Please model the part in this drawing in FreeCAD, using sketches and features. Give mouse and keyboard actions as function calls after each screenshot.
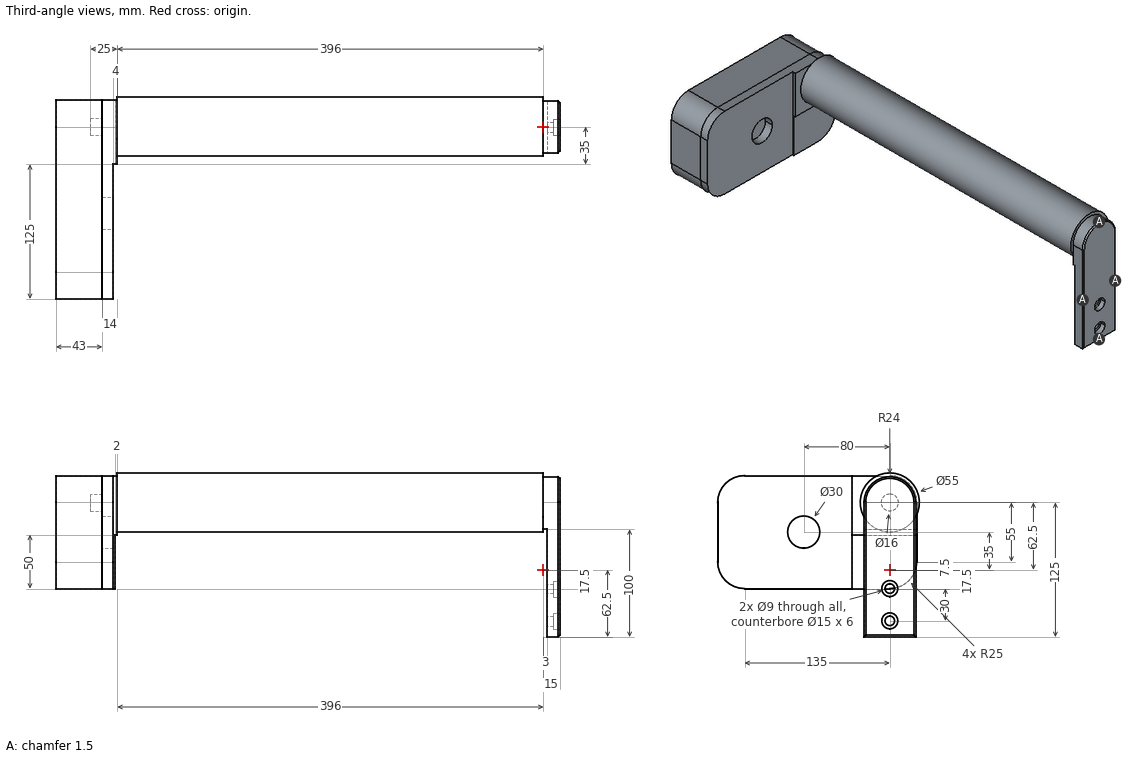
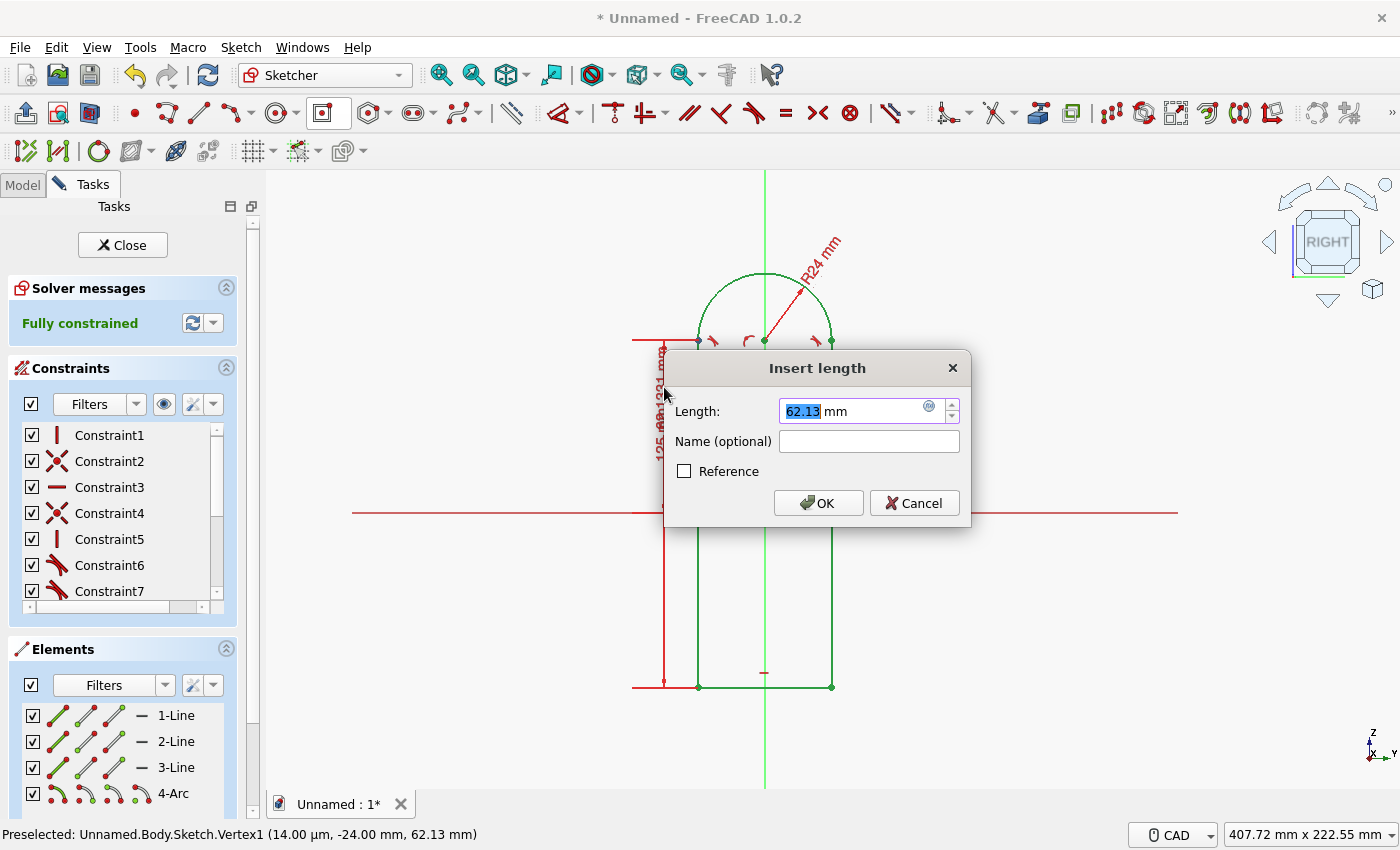
text(62.5)
key(Return)
key(Escape)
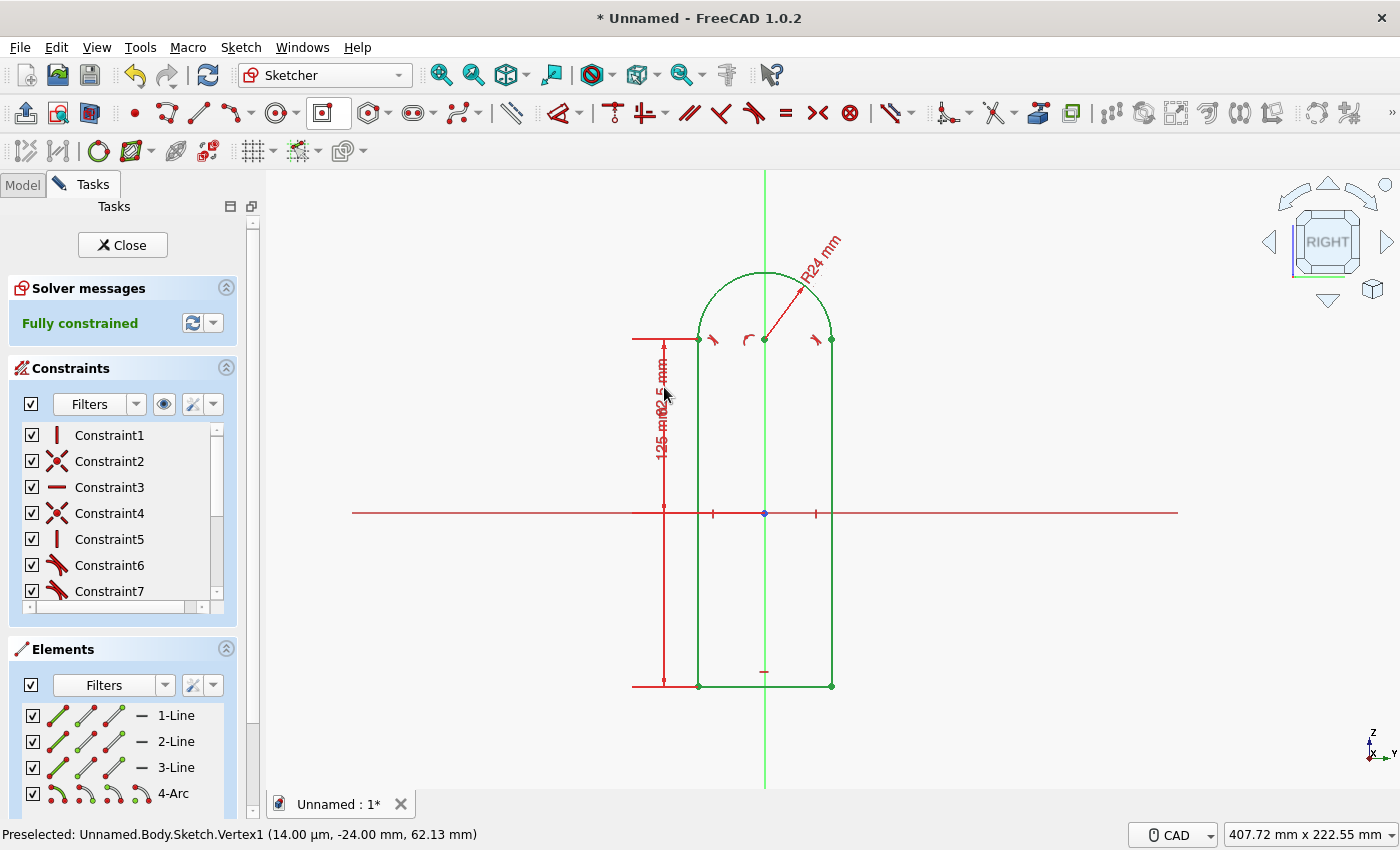
click(123, 245)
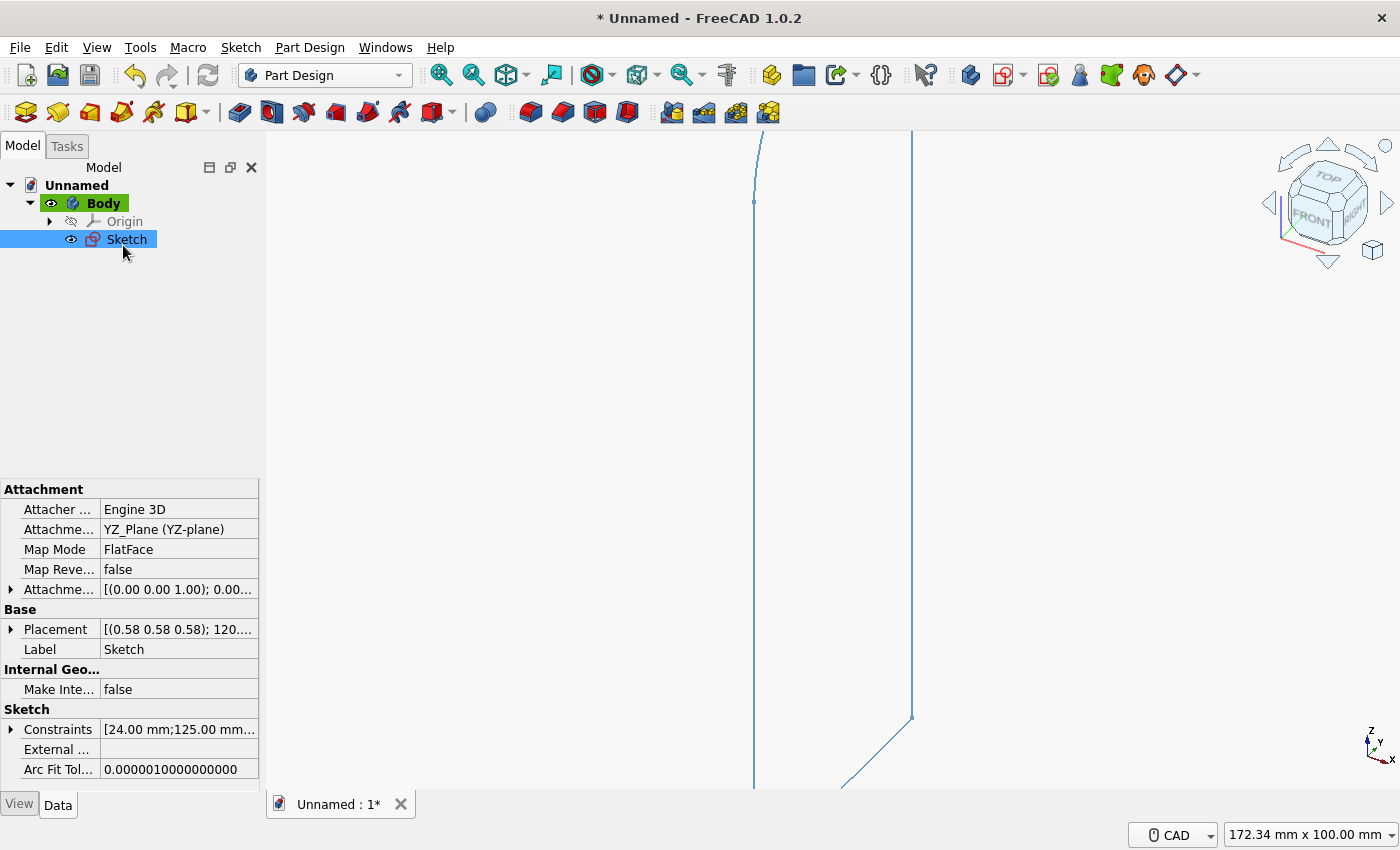
click(26, 112)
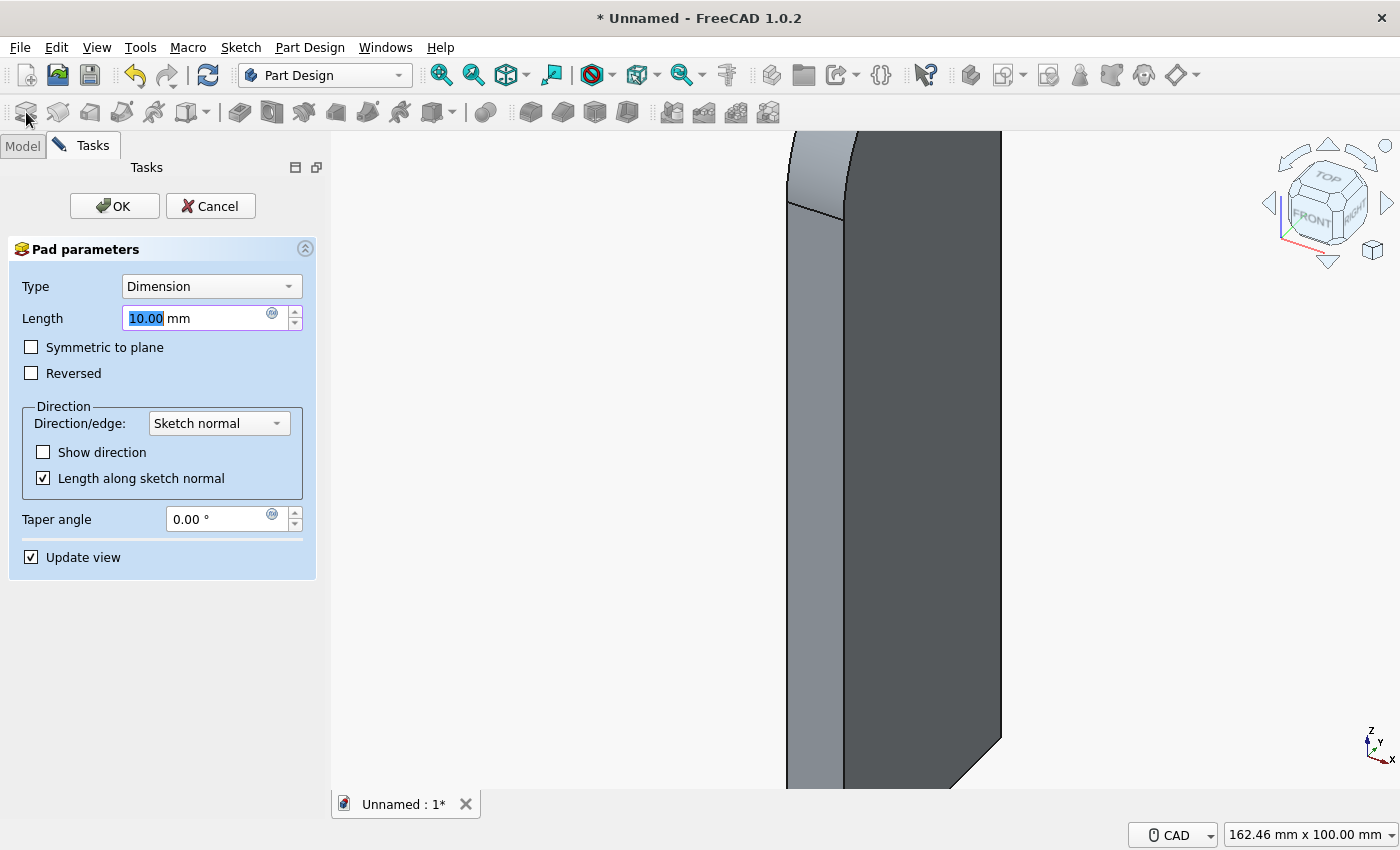
text(15)
key(Tab)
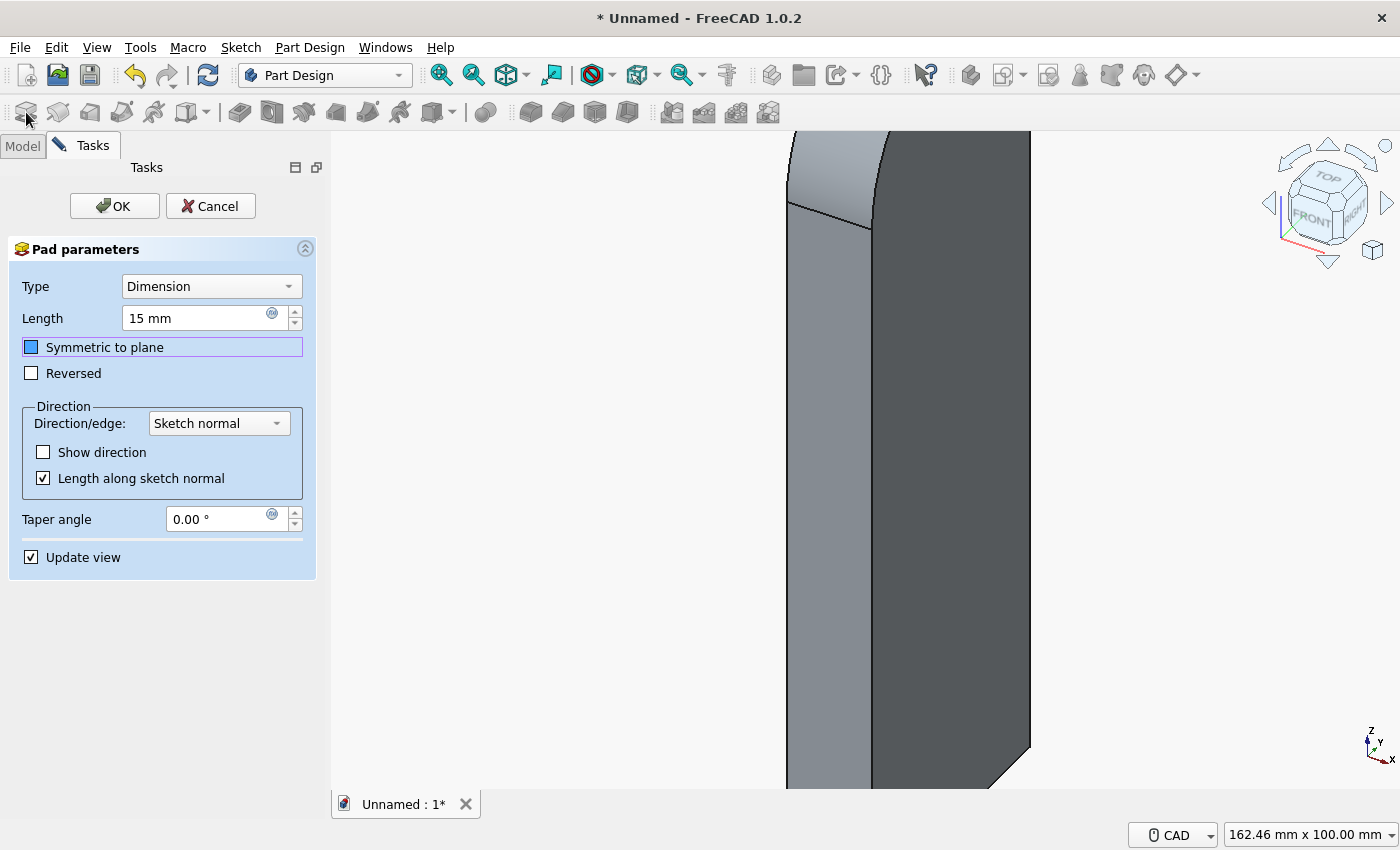
click(115, 206)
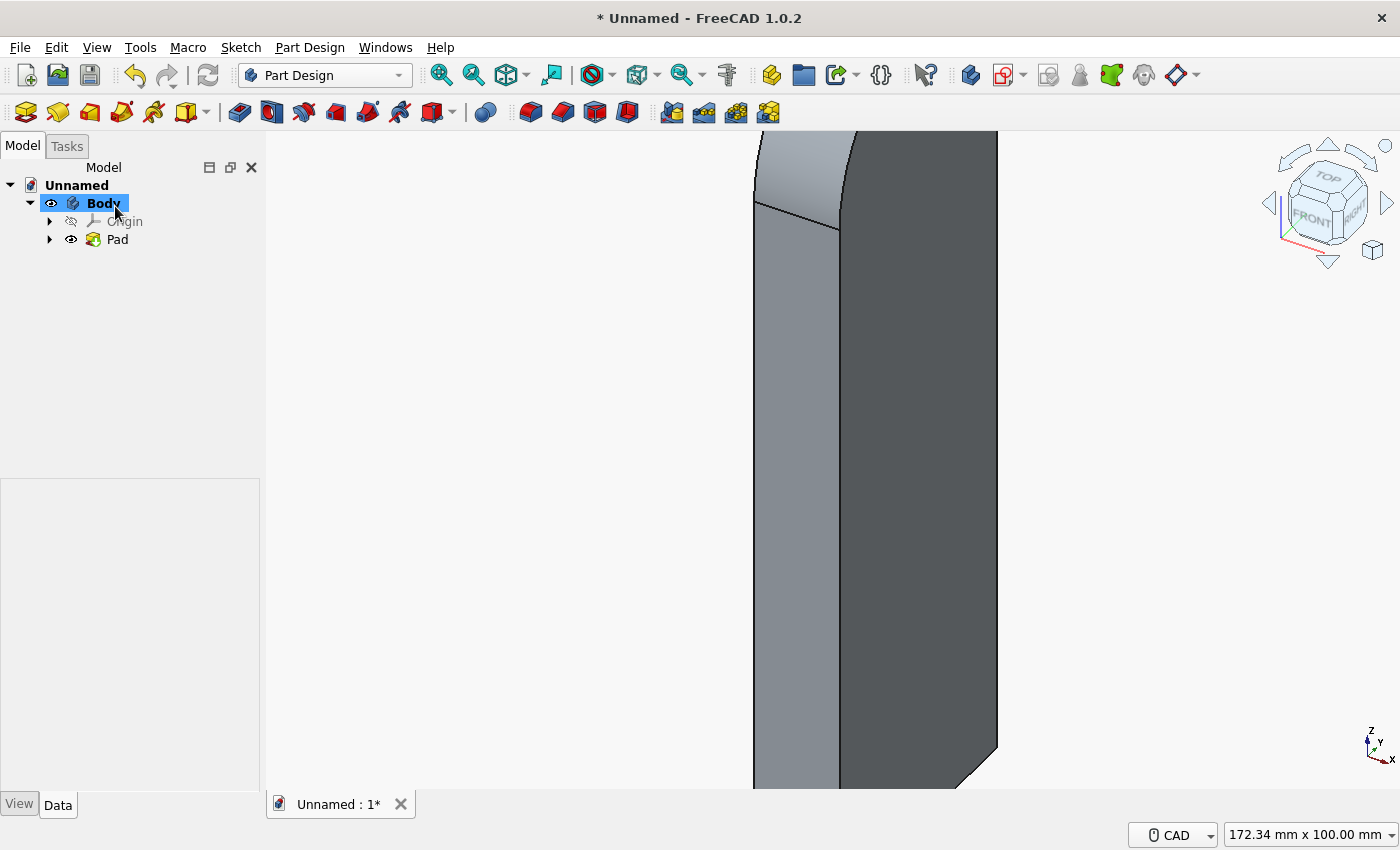
key(v)
key(f)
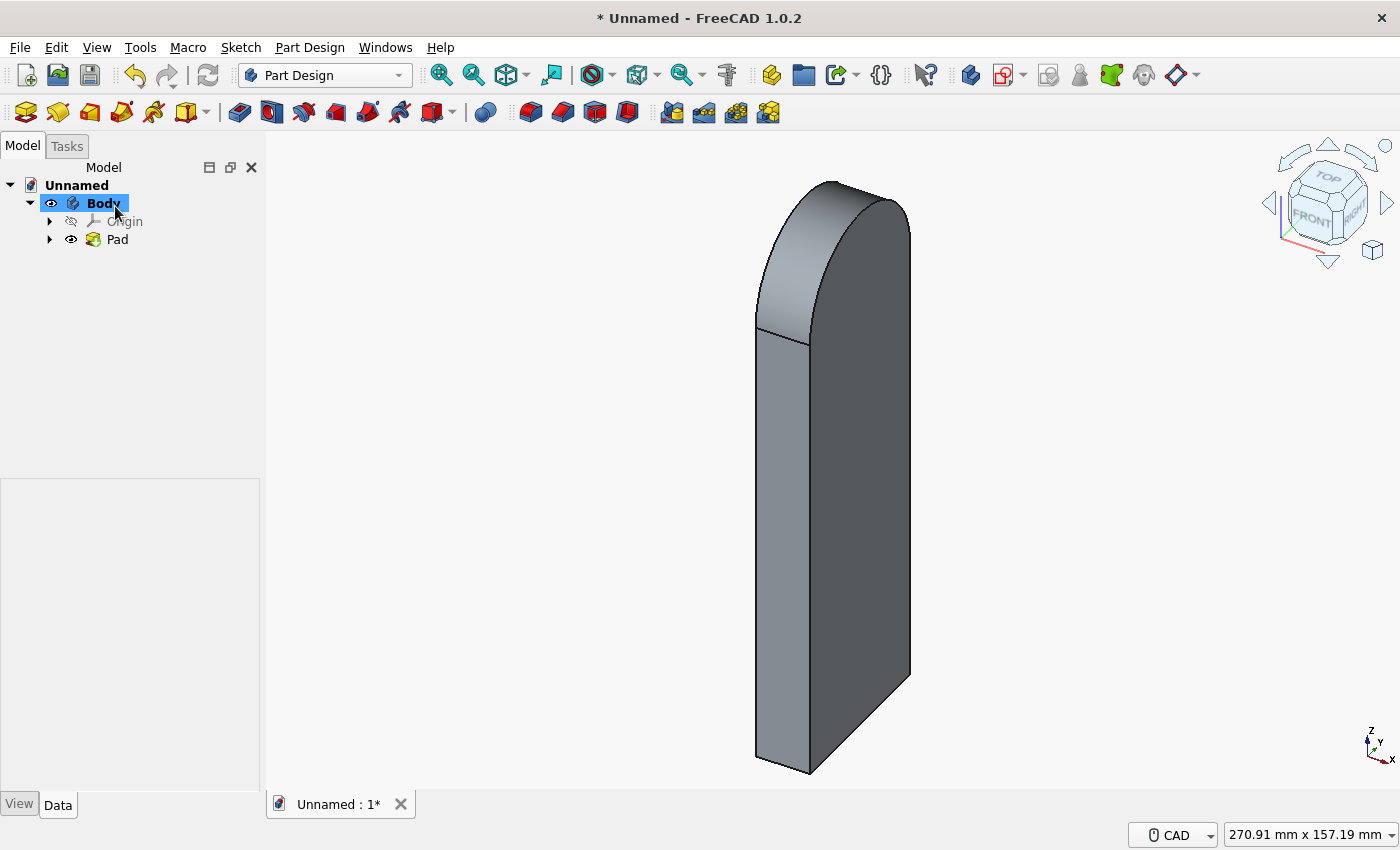
key(6)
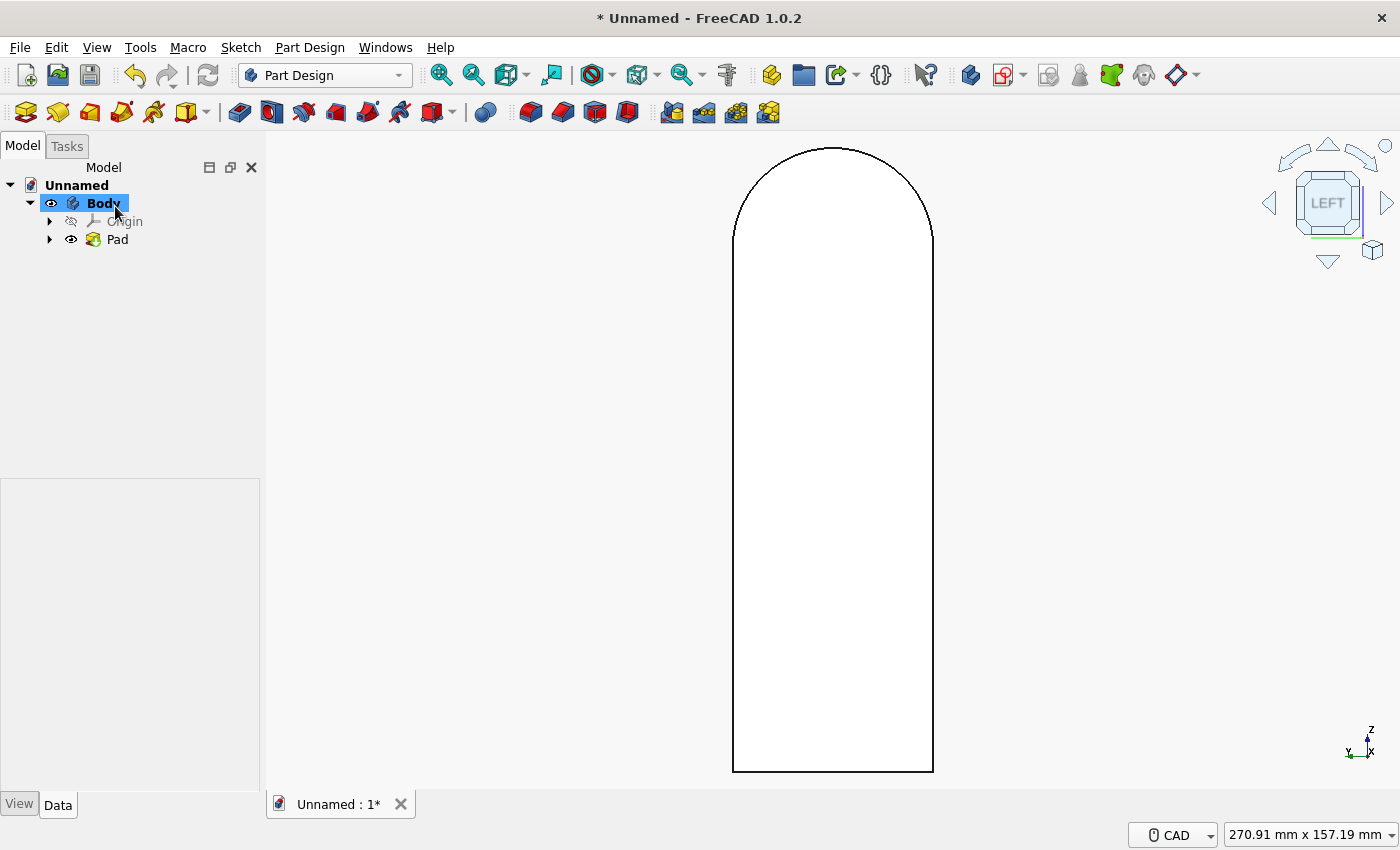
click(833, 637)